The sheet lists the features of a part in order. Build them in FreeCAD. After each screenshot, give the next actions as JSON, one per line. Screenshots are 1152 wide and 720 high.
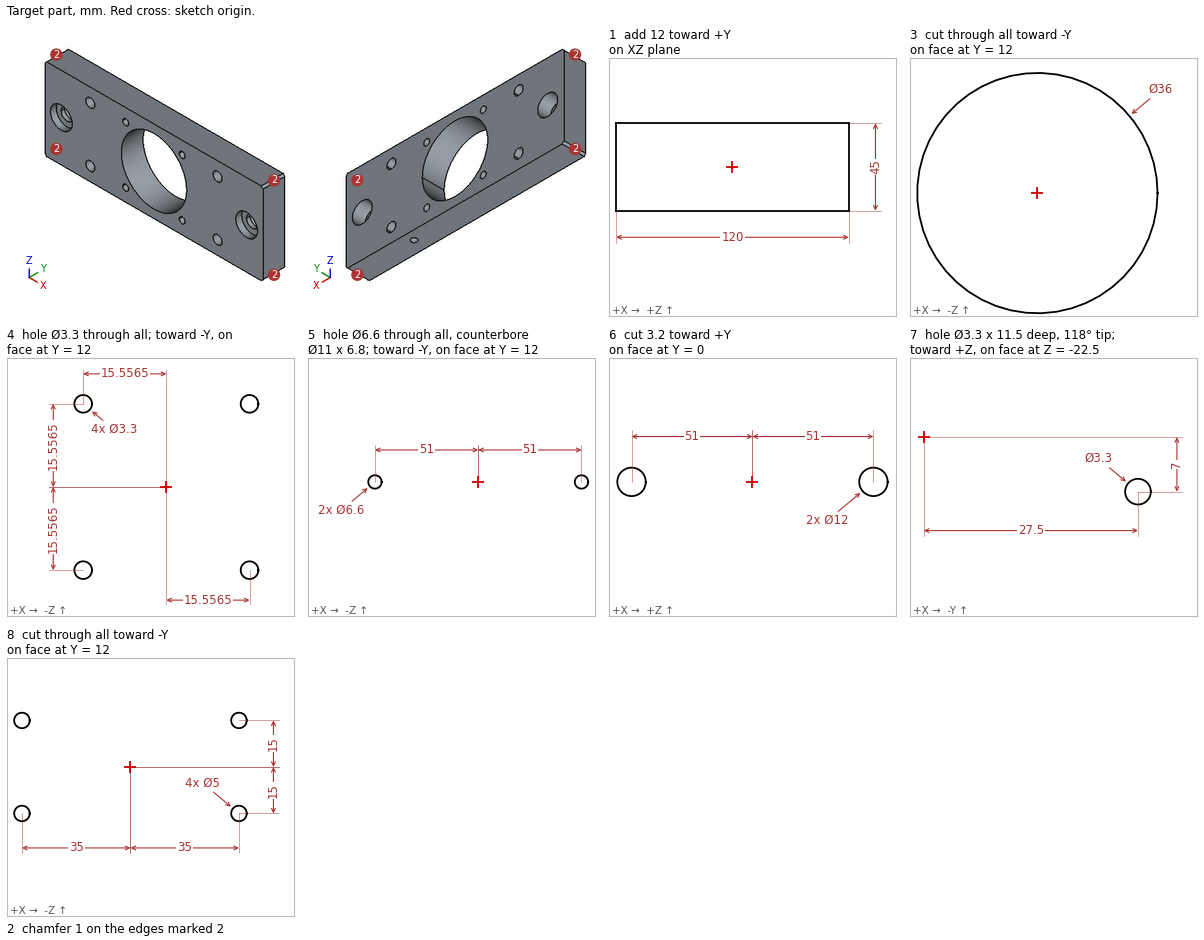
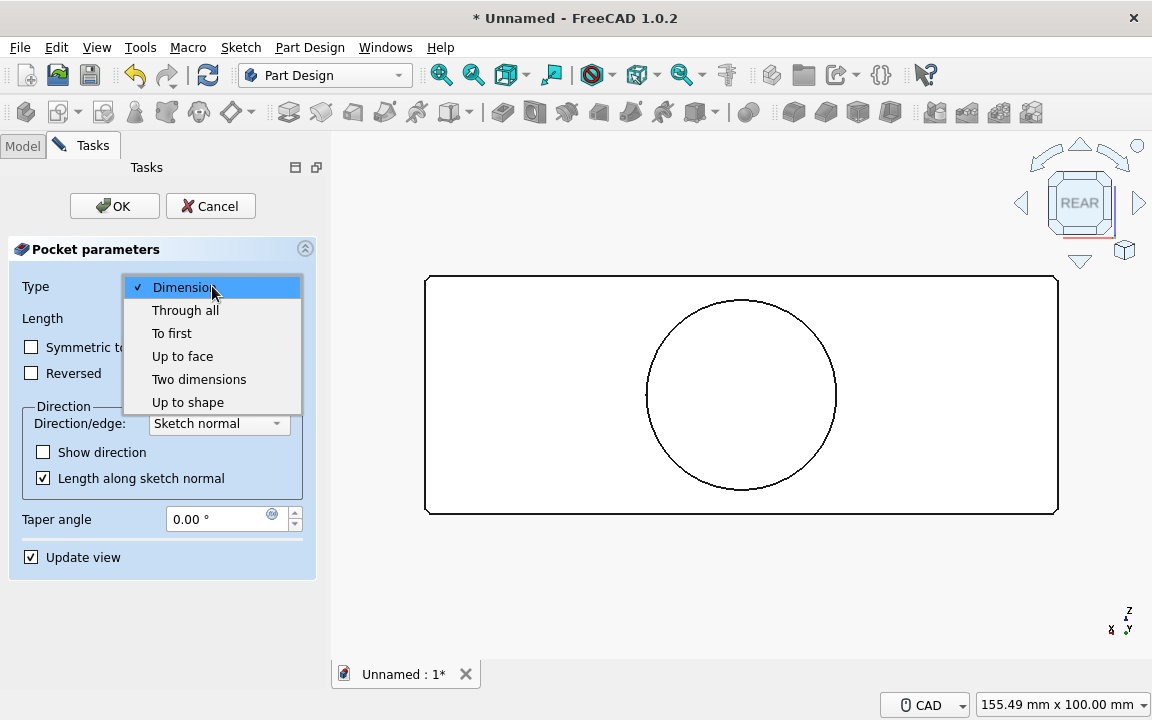
{"action": "left_click", "coordinate": [212, 310]}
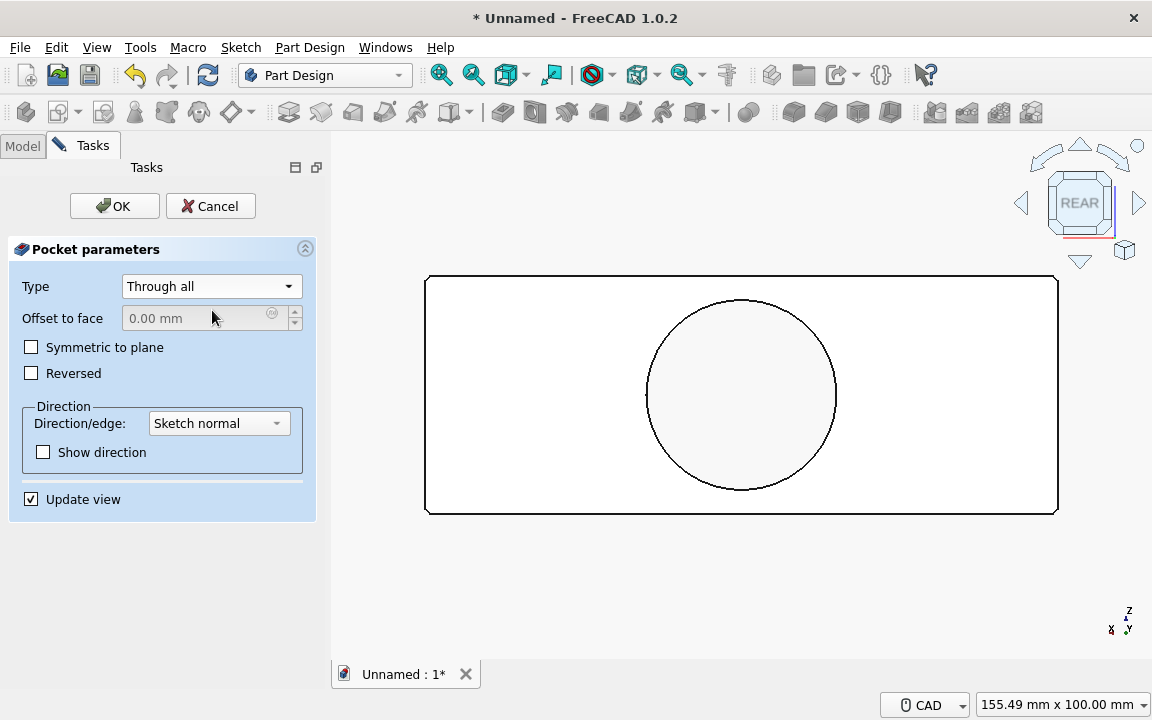
{"action": "left_click", "coordinate": [115, 206]}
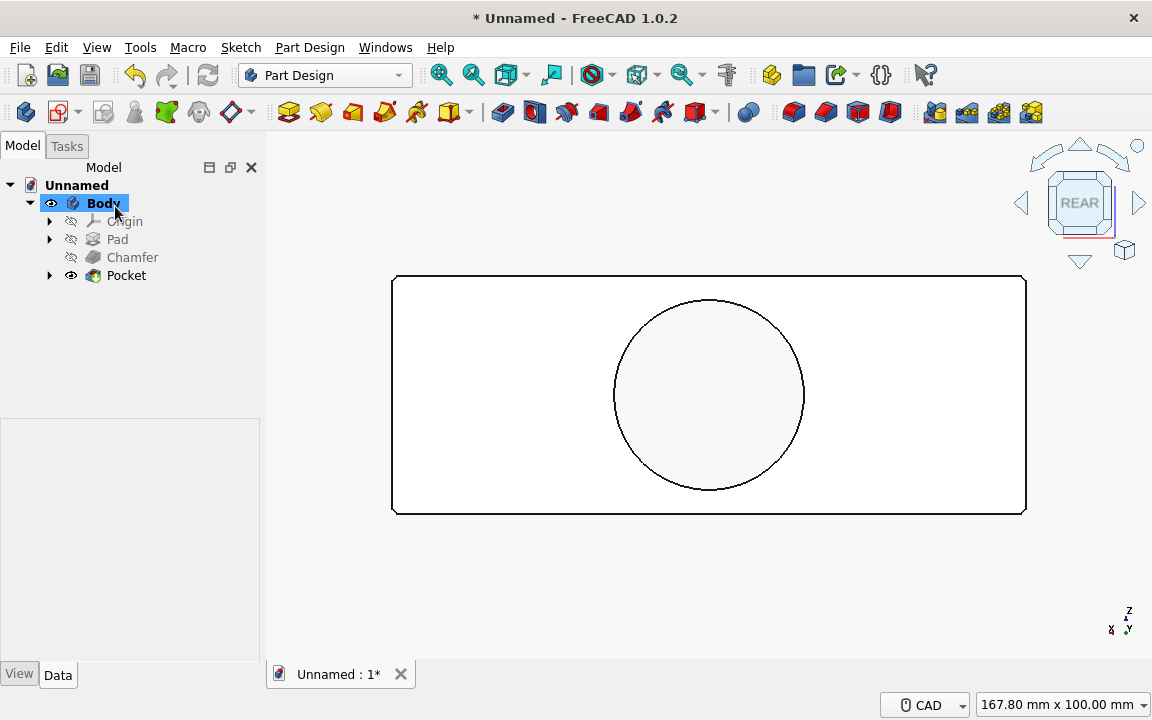
{"action": "left_click", "coordinate": [528, 394]}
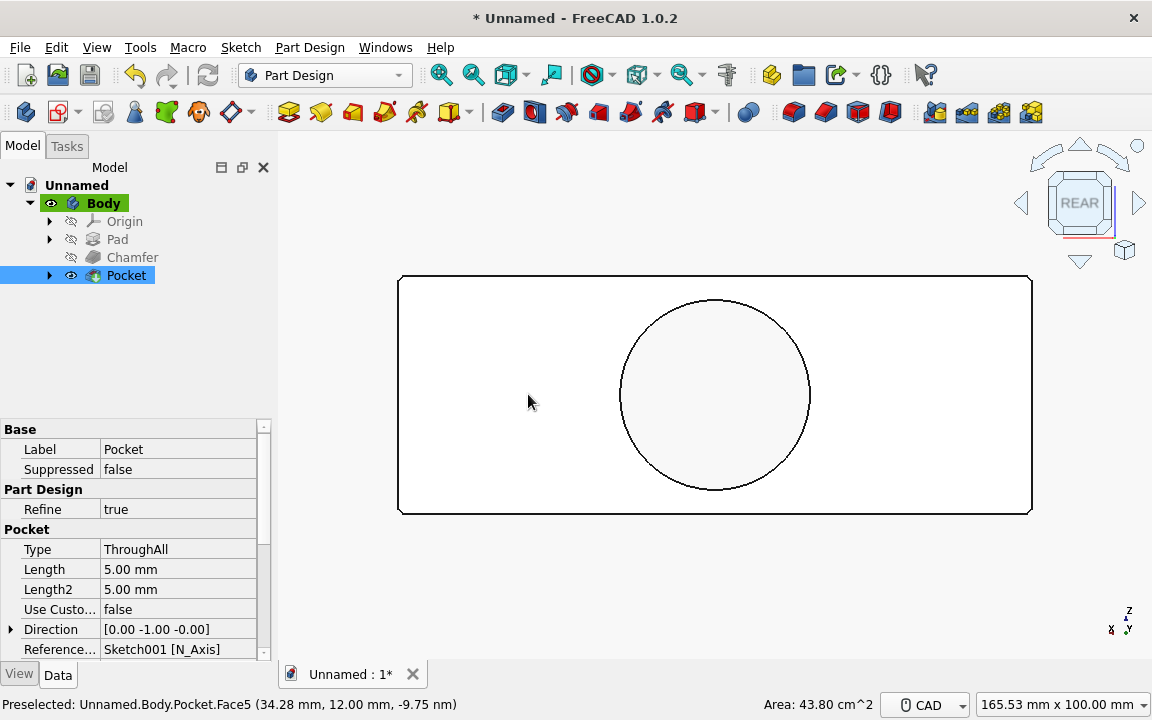
{"action": "left_click", "coordinate": [58, 112]}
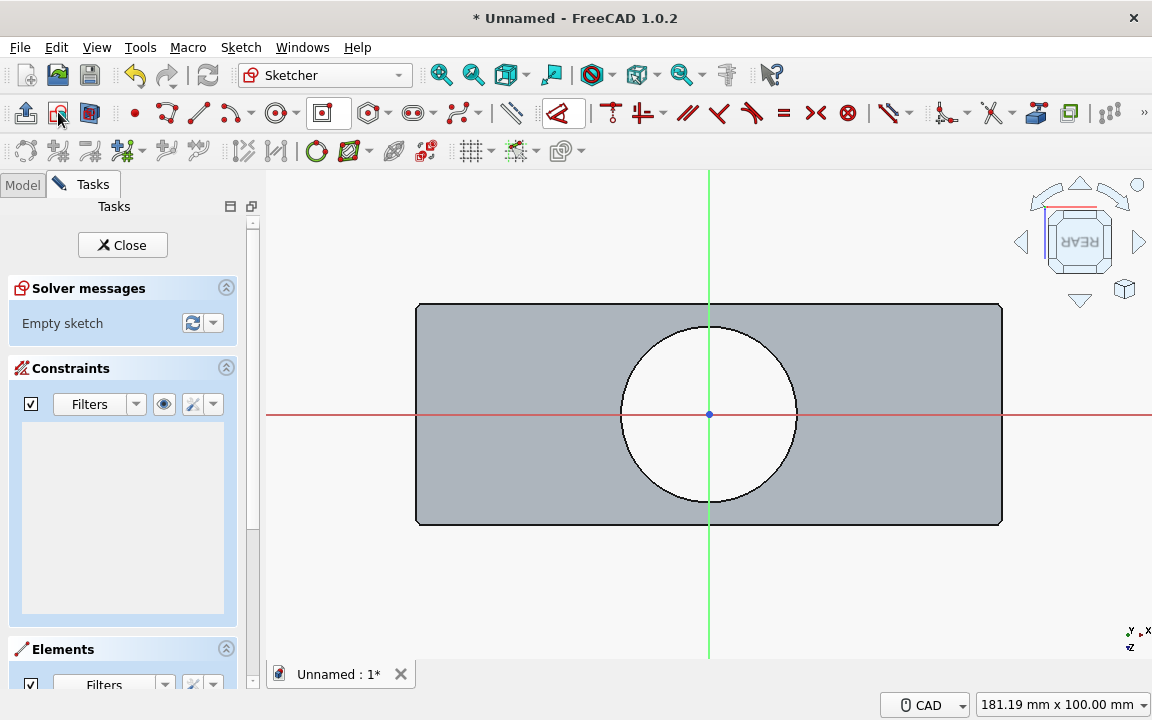
{"action": "scroll", "coordinate": [792, 414], "scroll_direction": "up", "scroll_amount": 3}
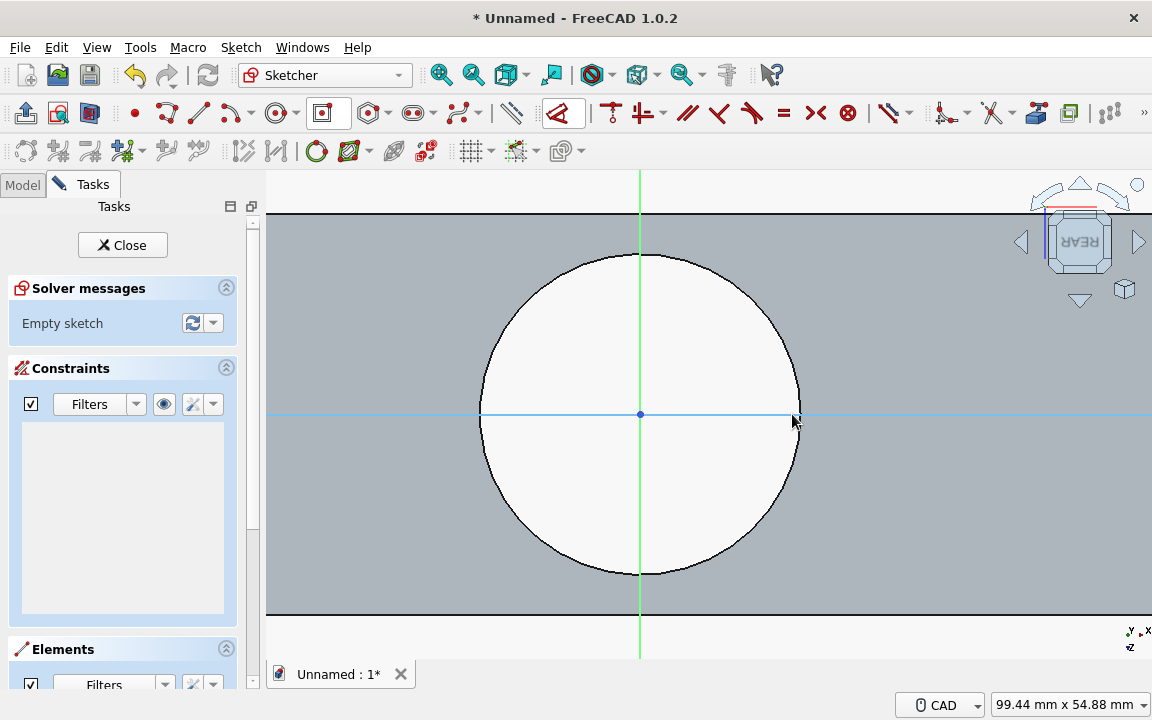
{"action": "left_click", "coordinate": [276, 114]}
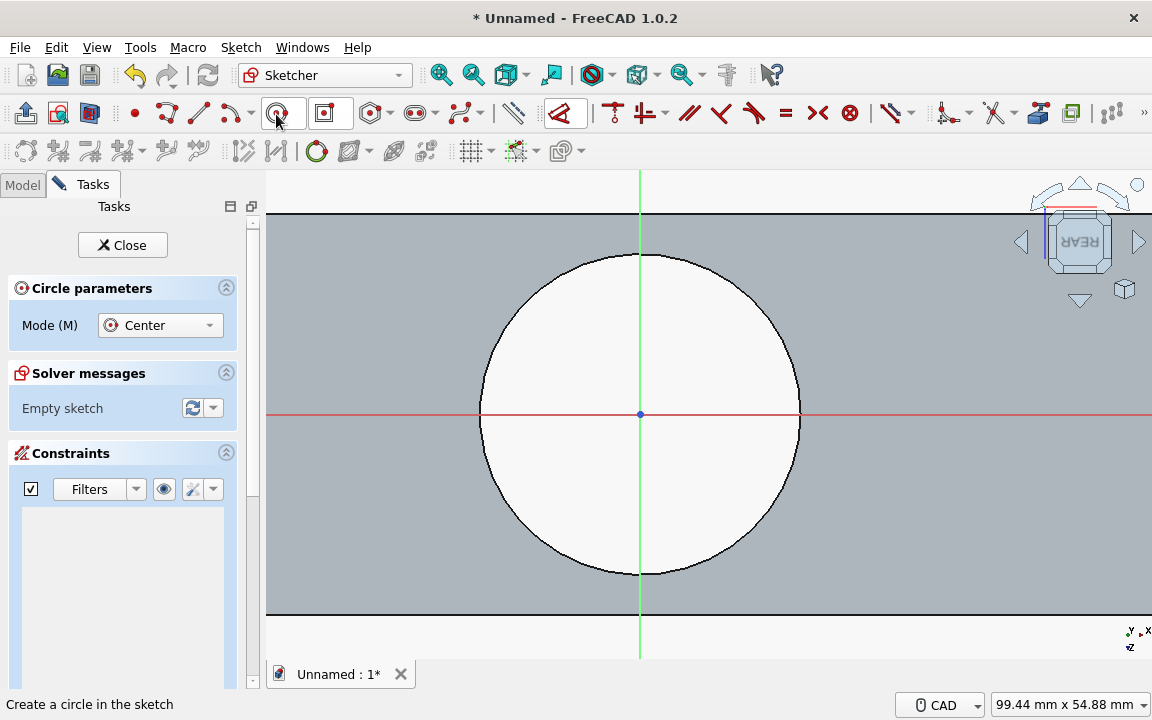
{"action": "scroll", "coordinate": [502, 276], "scroll_direction": "up", "scroll_amount": 3}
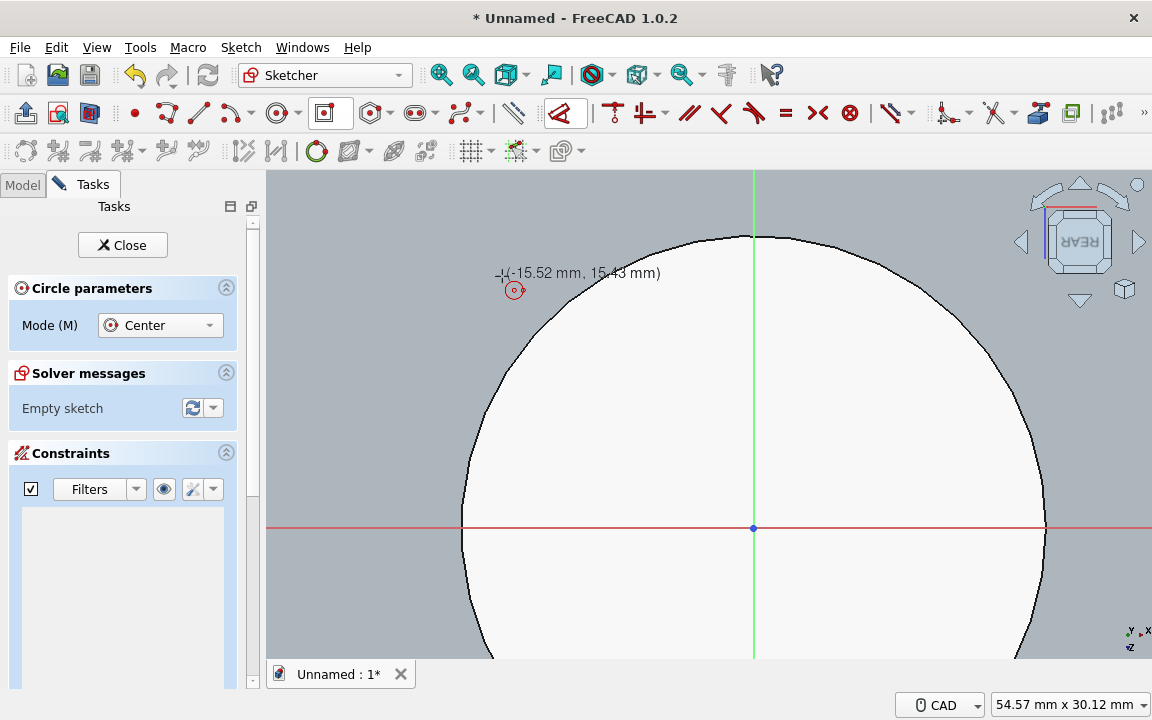
{"action": "left_click", "coordinate": [501, 276]}
{"action": "mouse_move", "coordinate": [520, 257]}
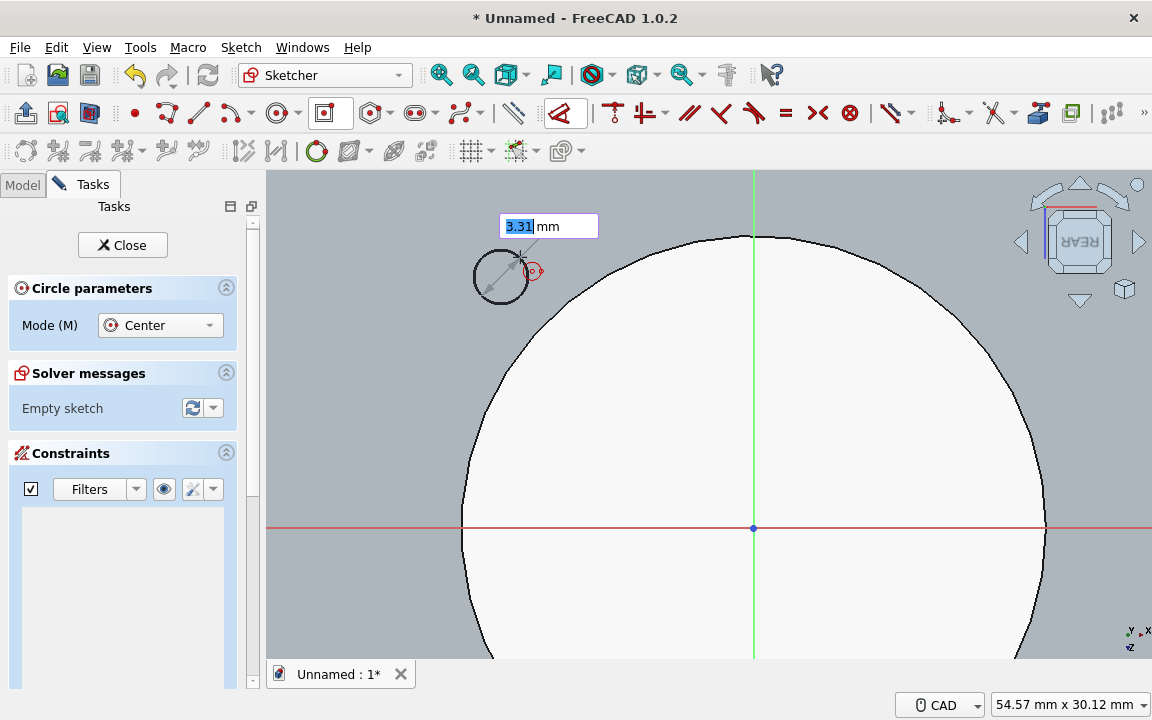
{"action": "type", "text": "3.3"}
{"action": "key", "text": "Return"}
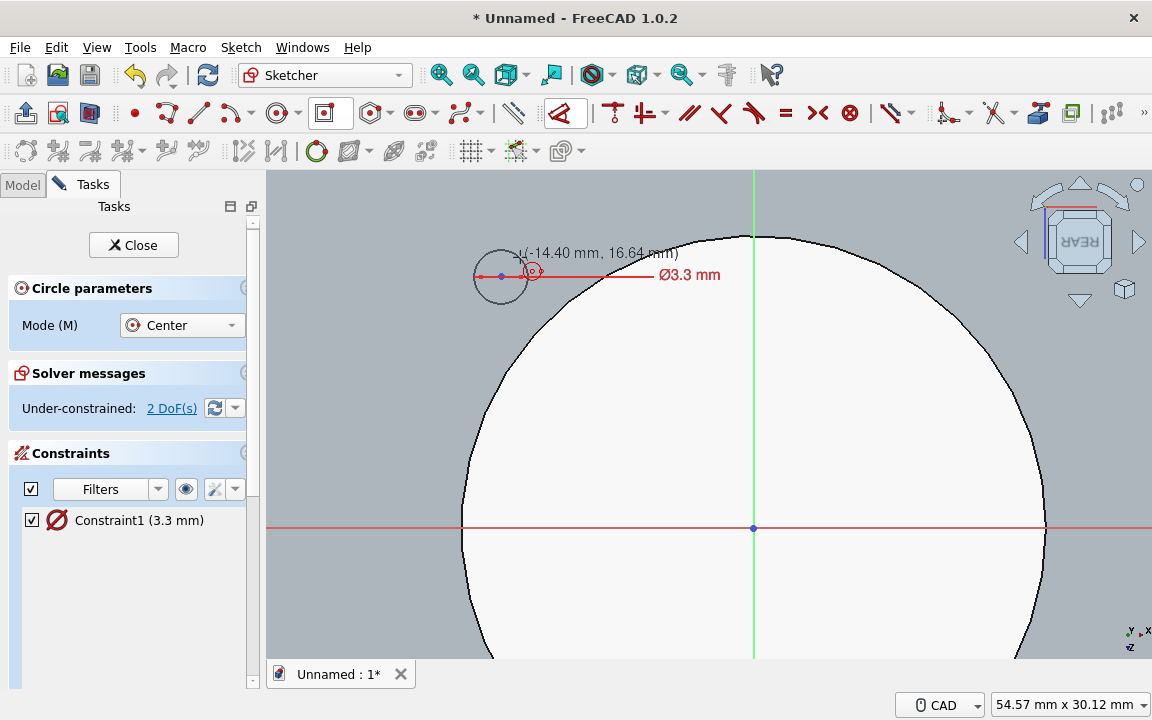
{"action": "scroll", "coordinate": [503, 276], "scroll_direction": "down", "scroll_amount": 3}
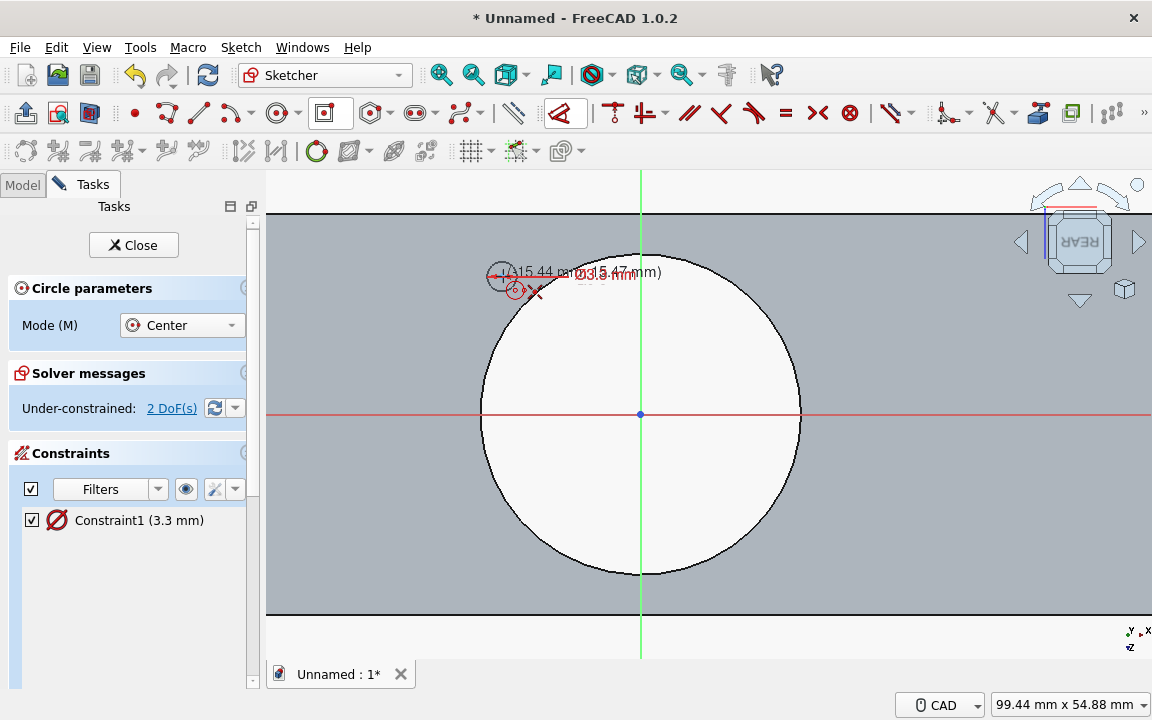
{"action": "scroll", "coordinate": [502, 553], "scroll_direction": "up", "scroll_amount": 3}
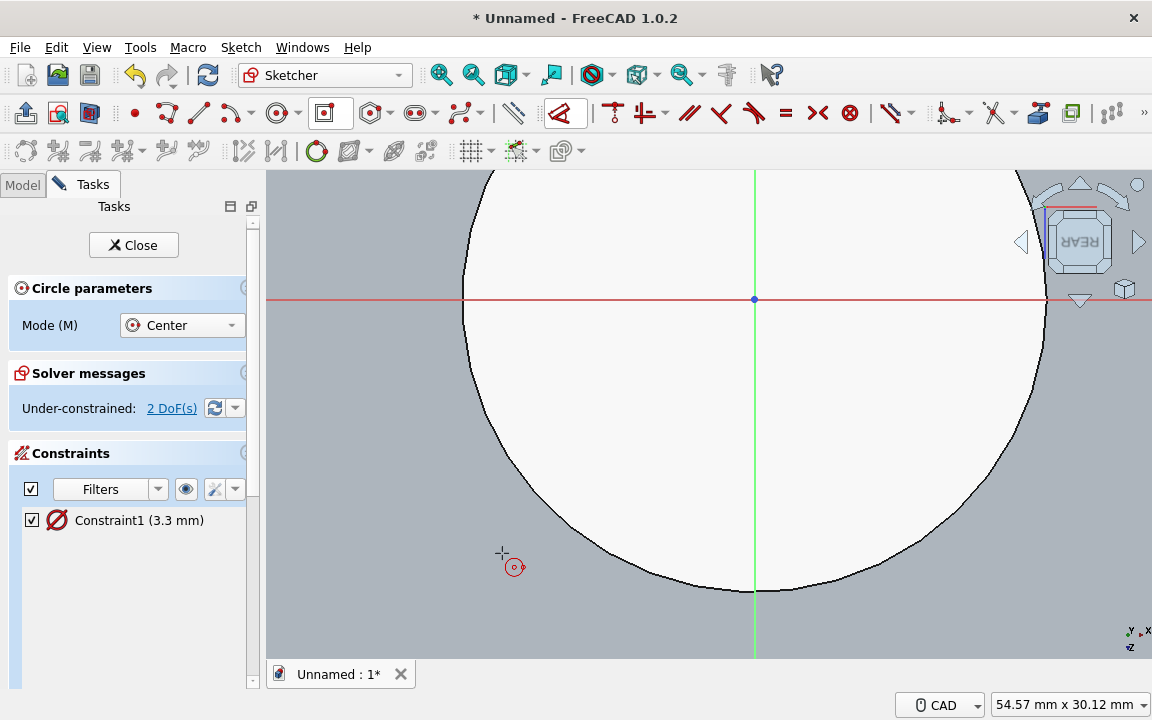
{"action": "left_click", "coordinate": [502, 553]}
{"action": "mouse_move", "coordinate": [521, 534]}